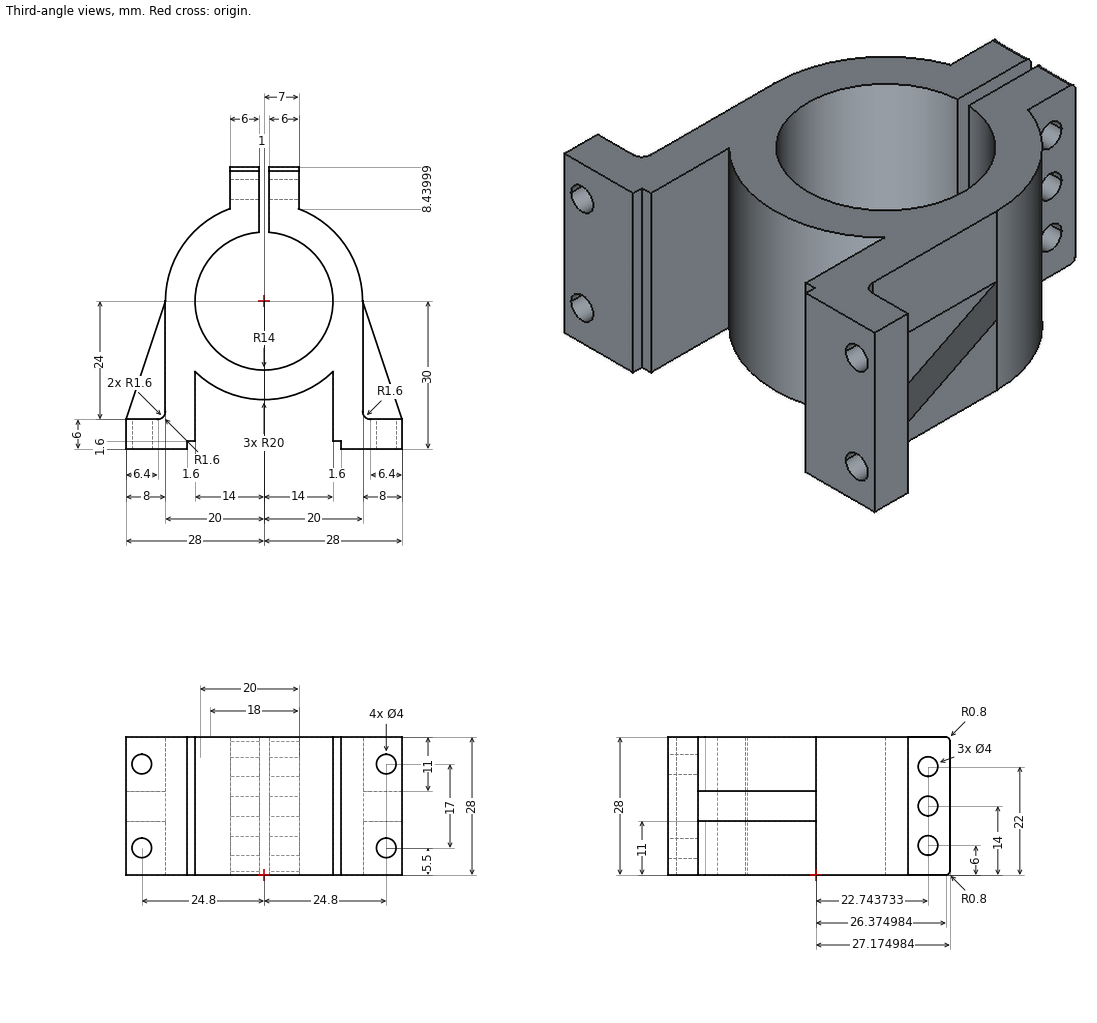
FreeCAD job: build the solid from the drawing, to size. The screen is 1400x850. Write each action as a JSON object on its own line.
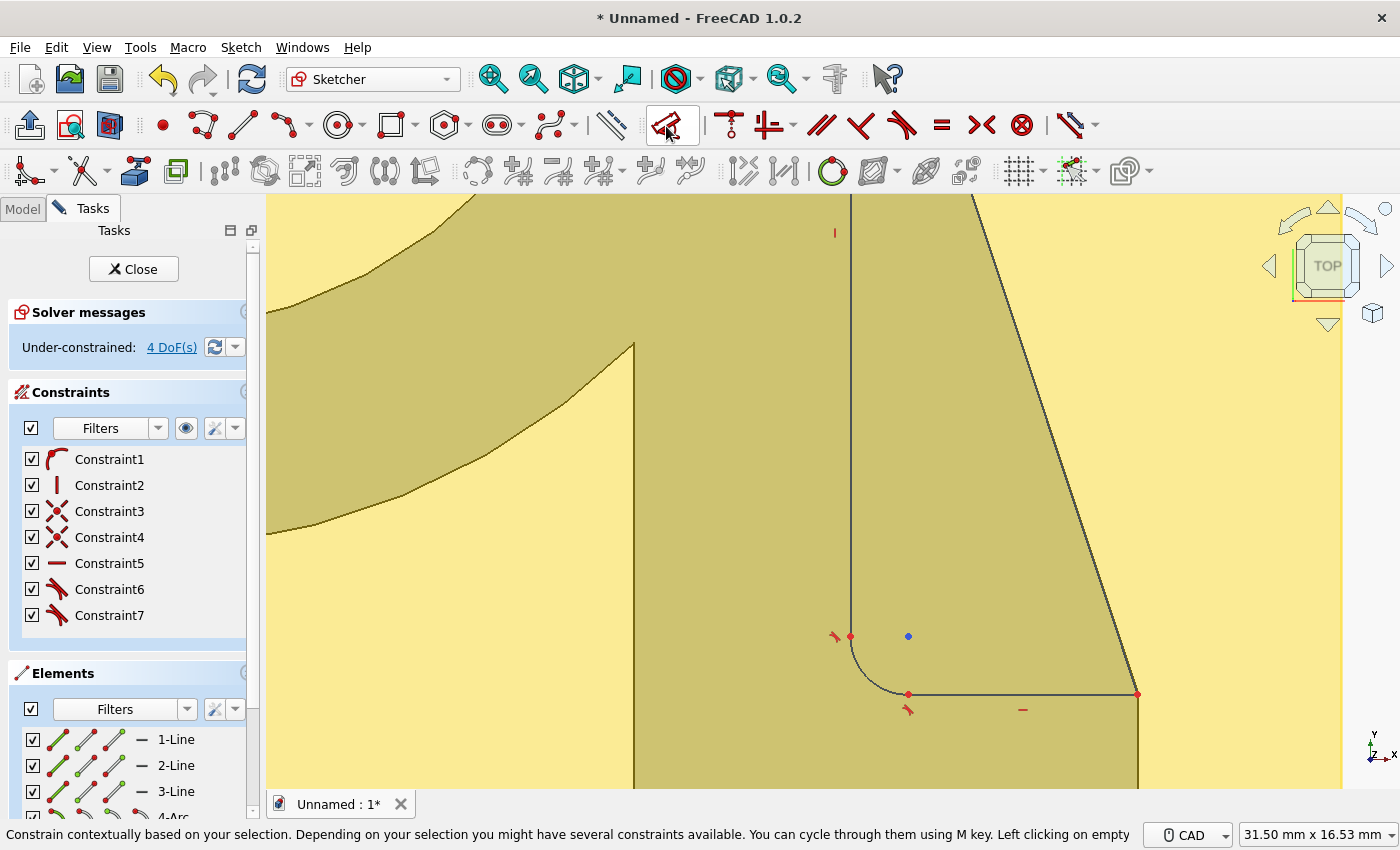
{"action": "left_click", "coordinate": [857, 663]}
{"action": "left_click", "coordinate": [828, 678]}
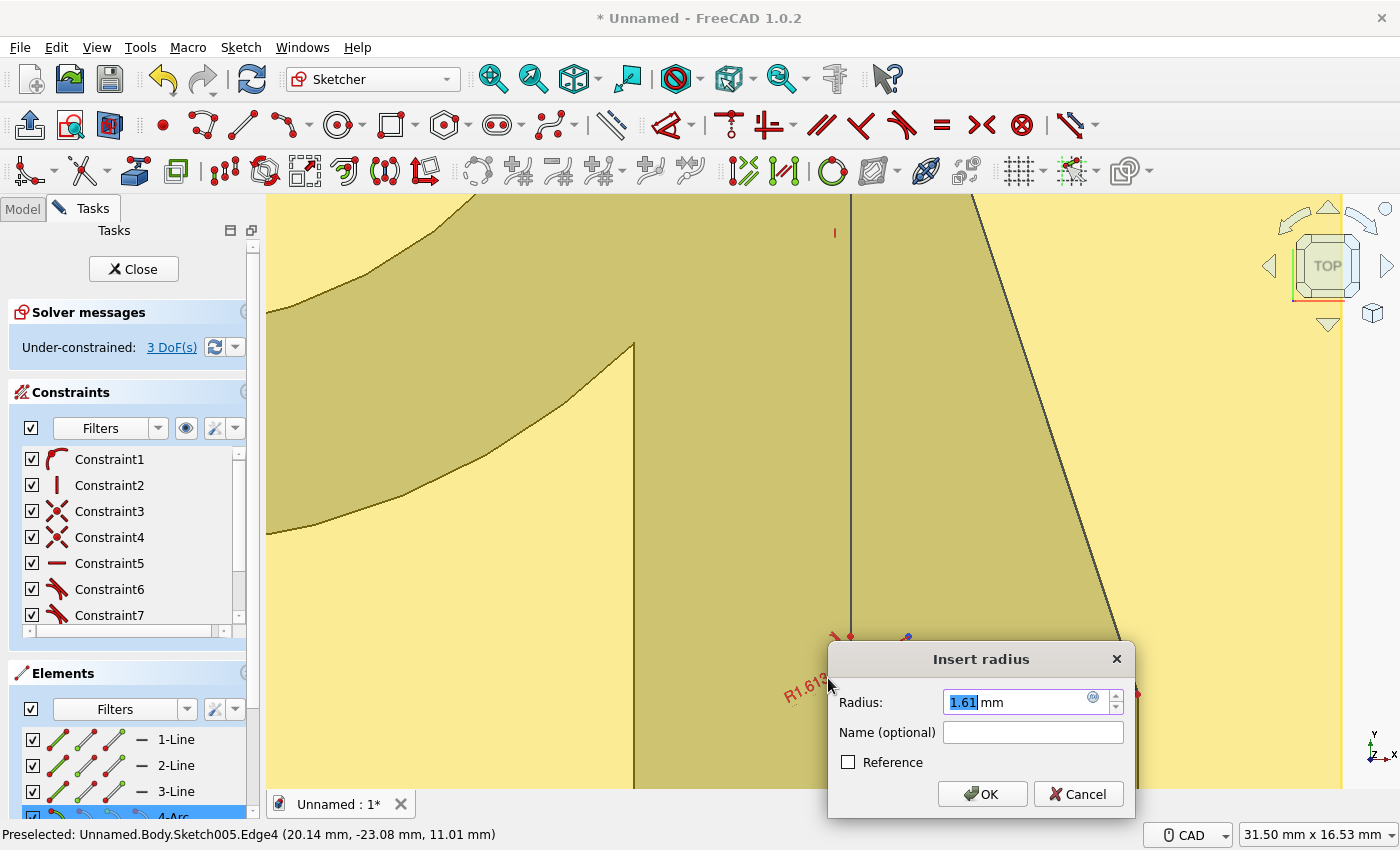
{"action": "type", "text": "1.6"}
{"action": "key", "text": "Return"}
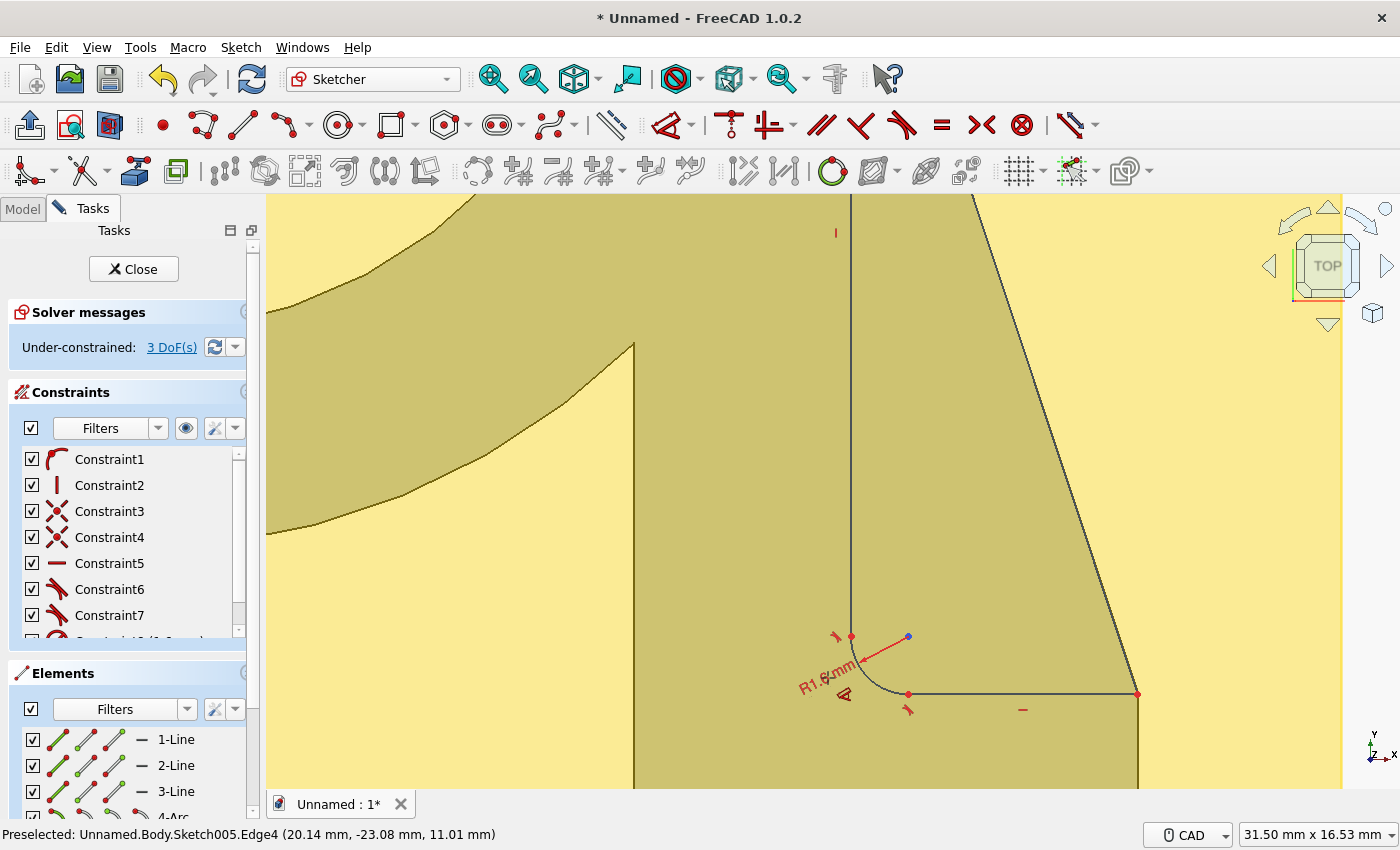
{"action": "left_click", "coordinate": [1052, 435]}
{"action": "left_click", "coordinate": [994, 728]}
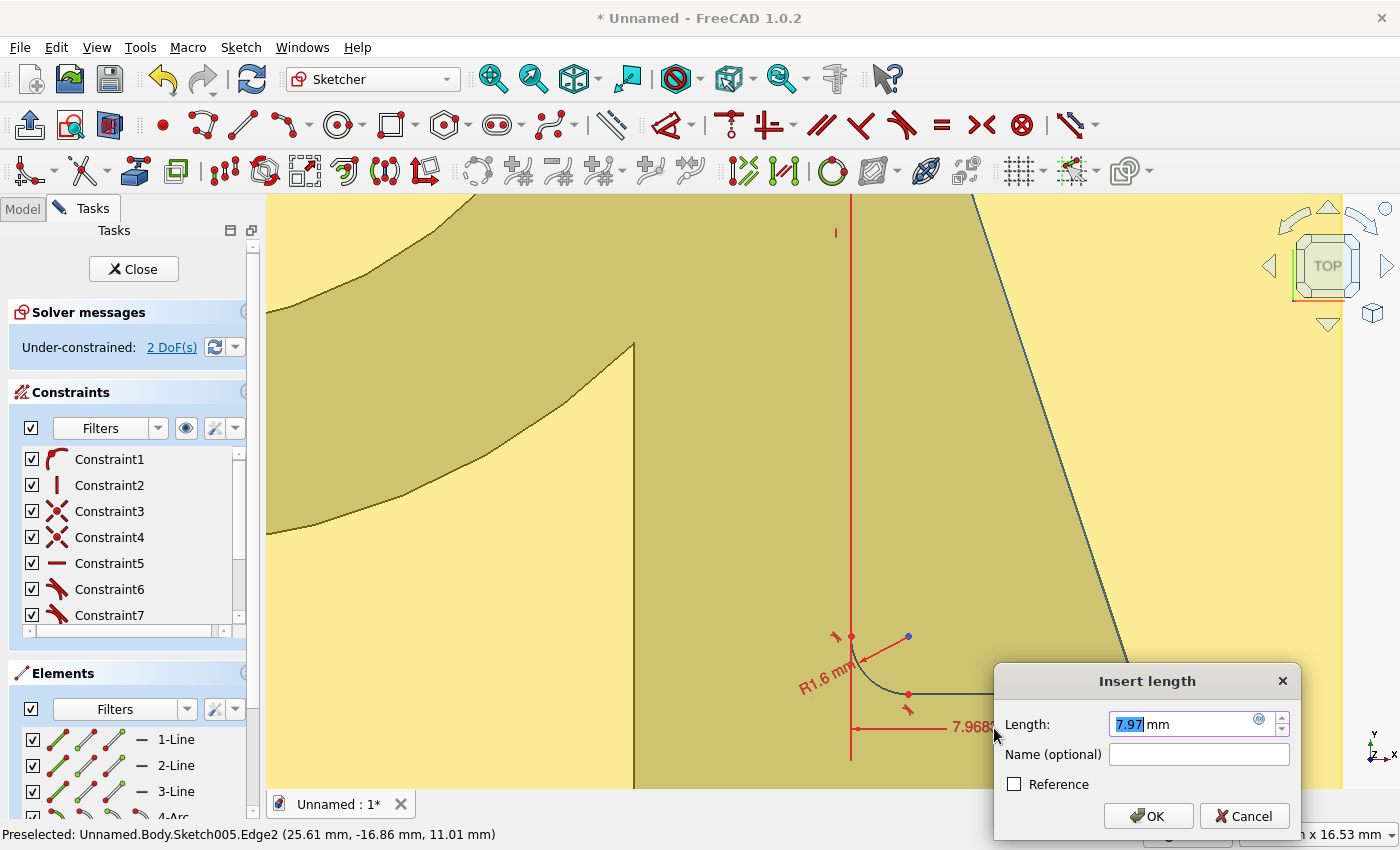
{"action": "type", "text": "8"}
{"action": "key", "text": "Return"}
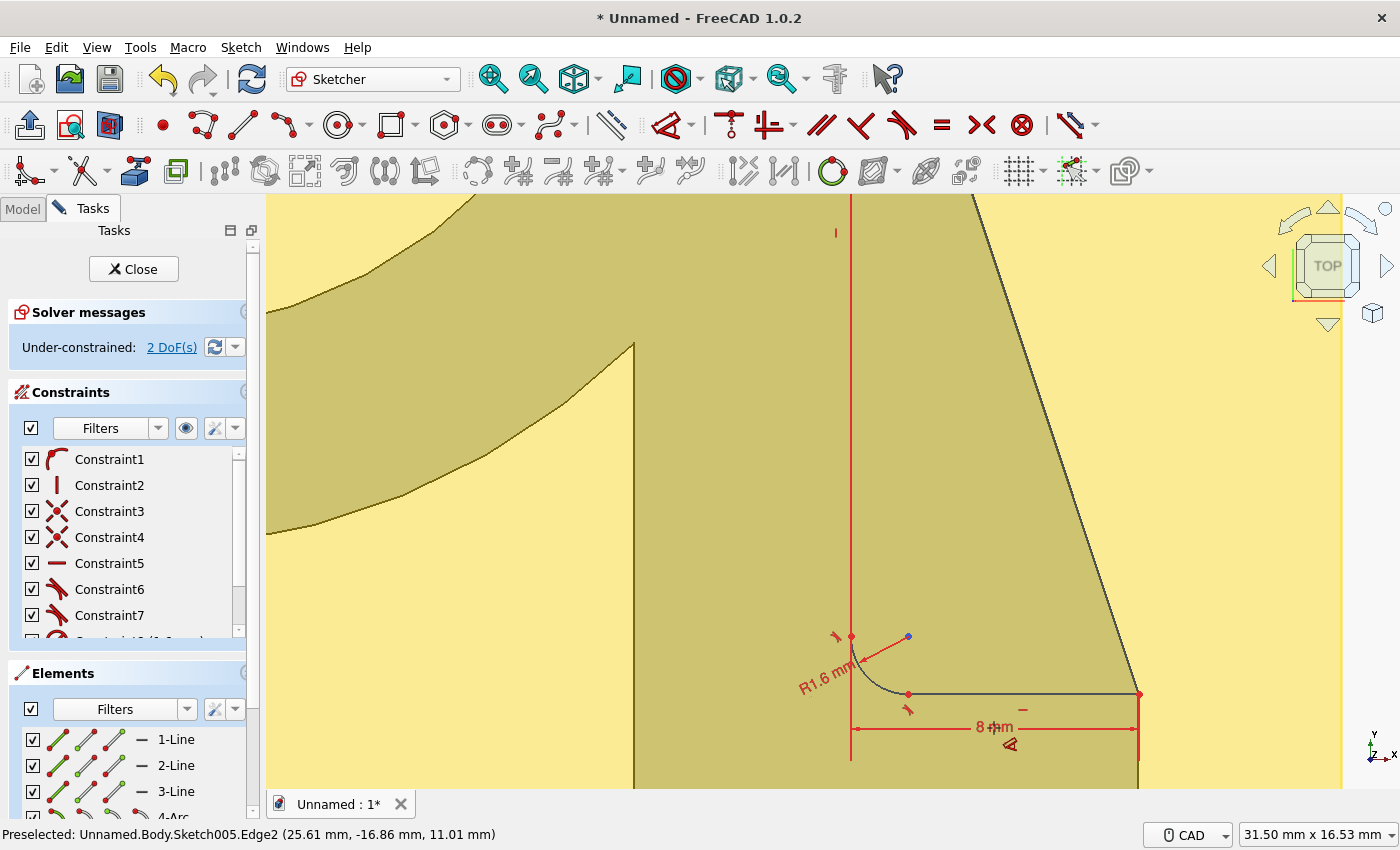
{"action": "left_click", "coordinate": [851, 637]}
{"action": "left_click", "coordinate": [573, 671]}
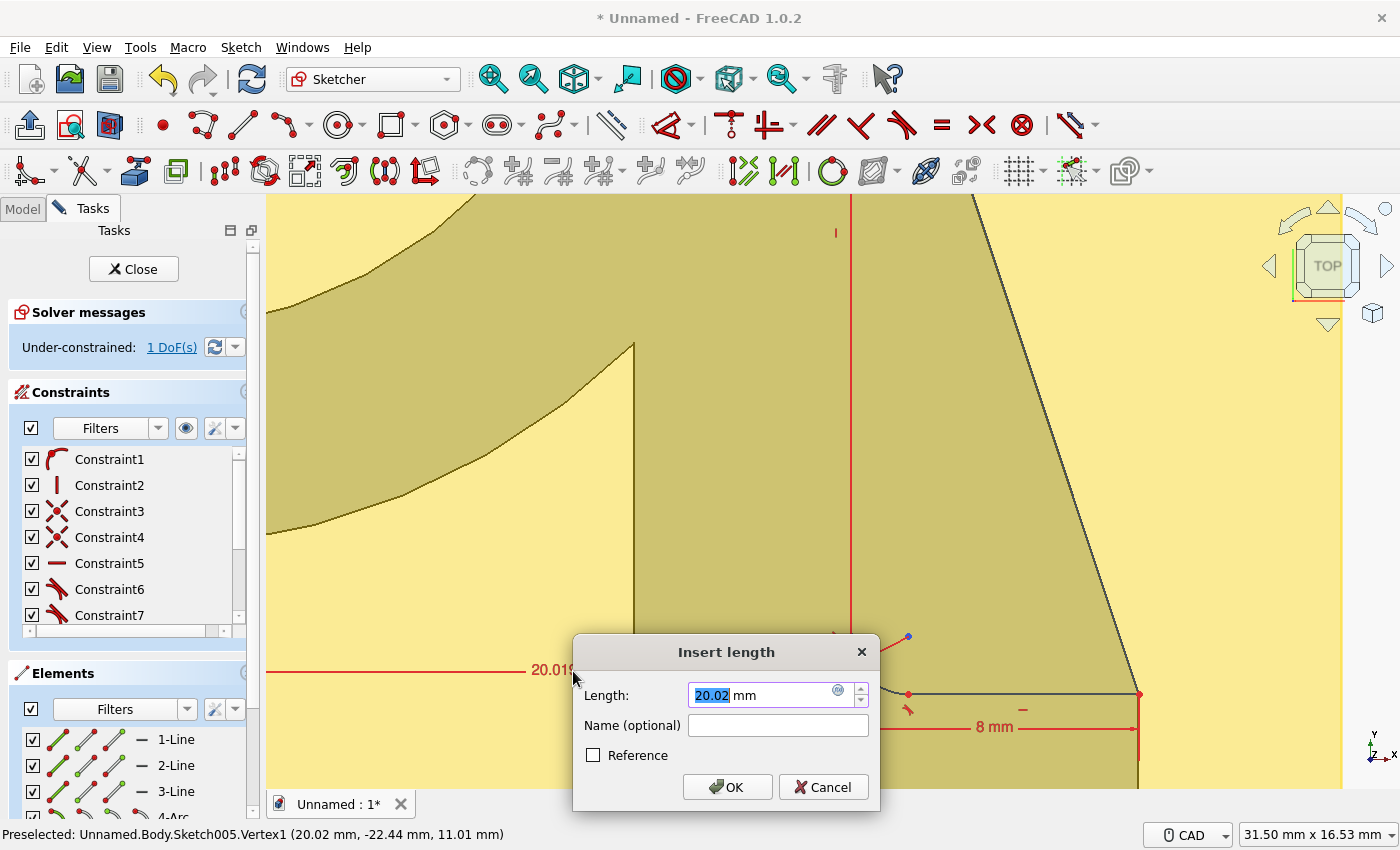
{"action": "type", "text": "20"}
{"action": "key", "text": "Return"}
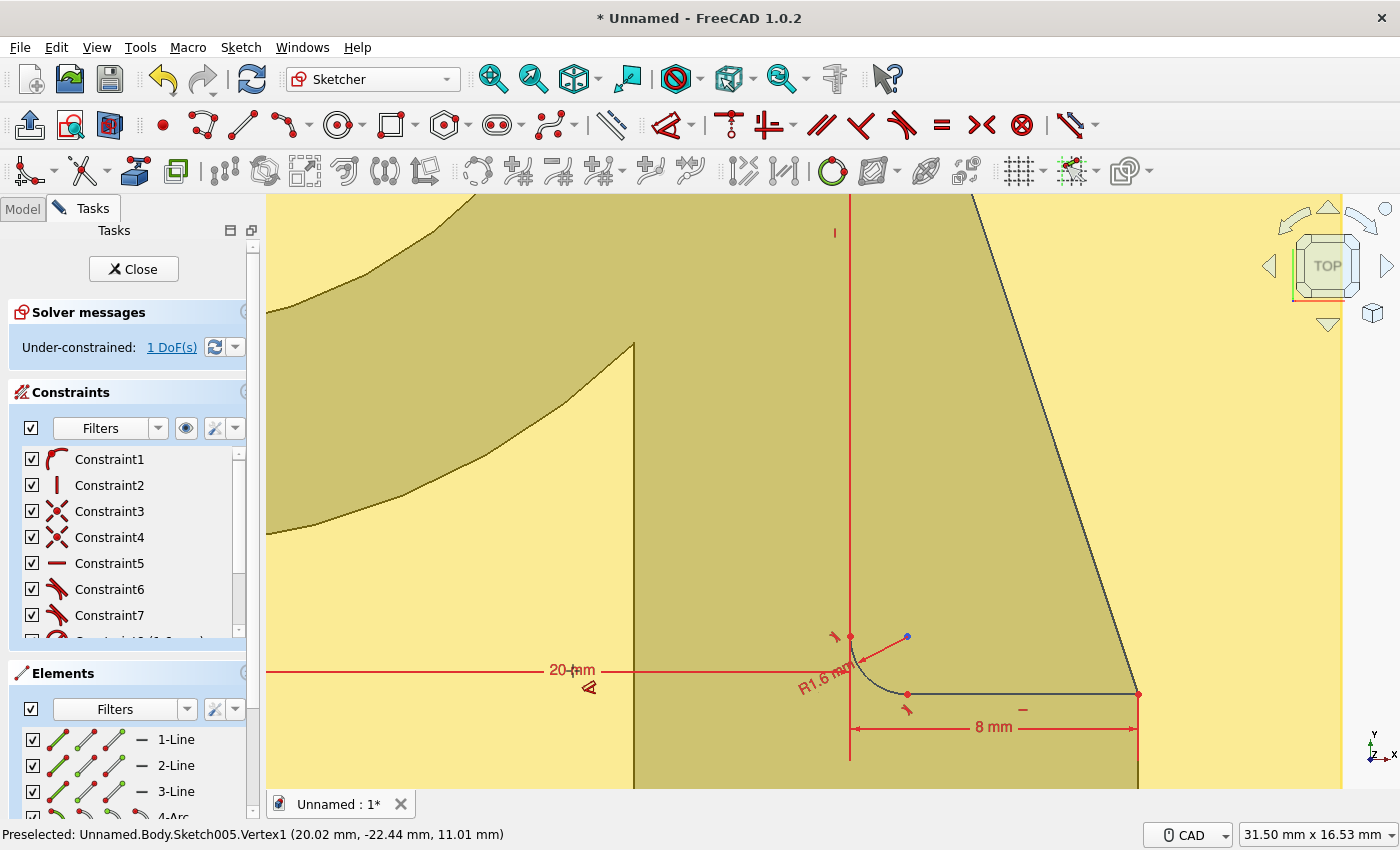
{"action": "left_click", "coordinate": [1138, 694]}
{"action": "left_click", "coordinate": [1172, 458]}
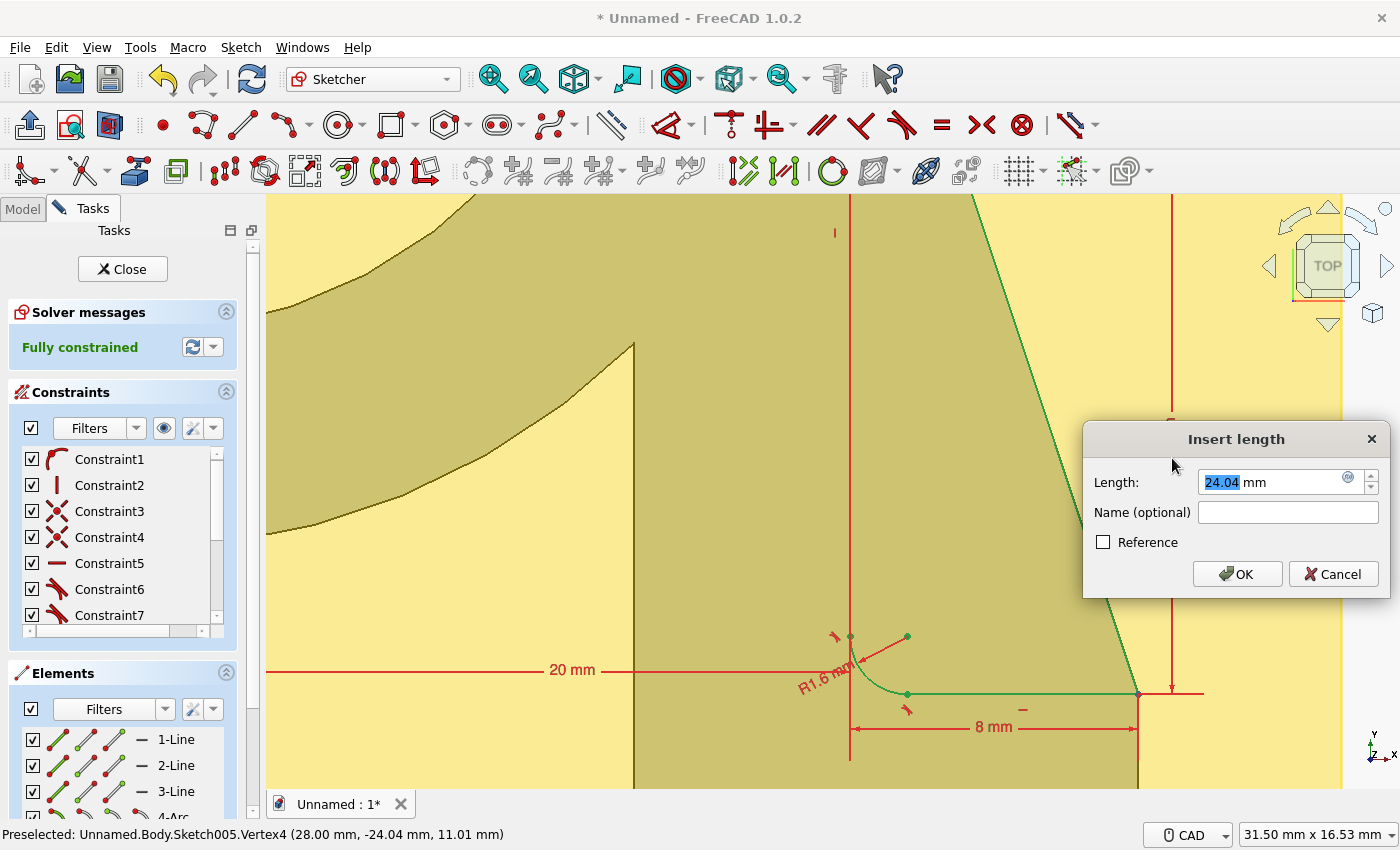
{"action": "type", "text": "24"}
{"action": "key", "text": "Return"}
{"action": "key", "text": "Escape"}